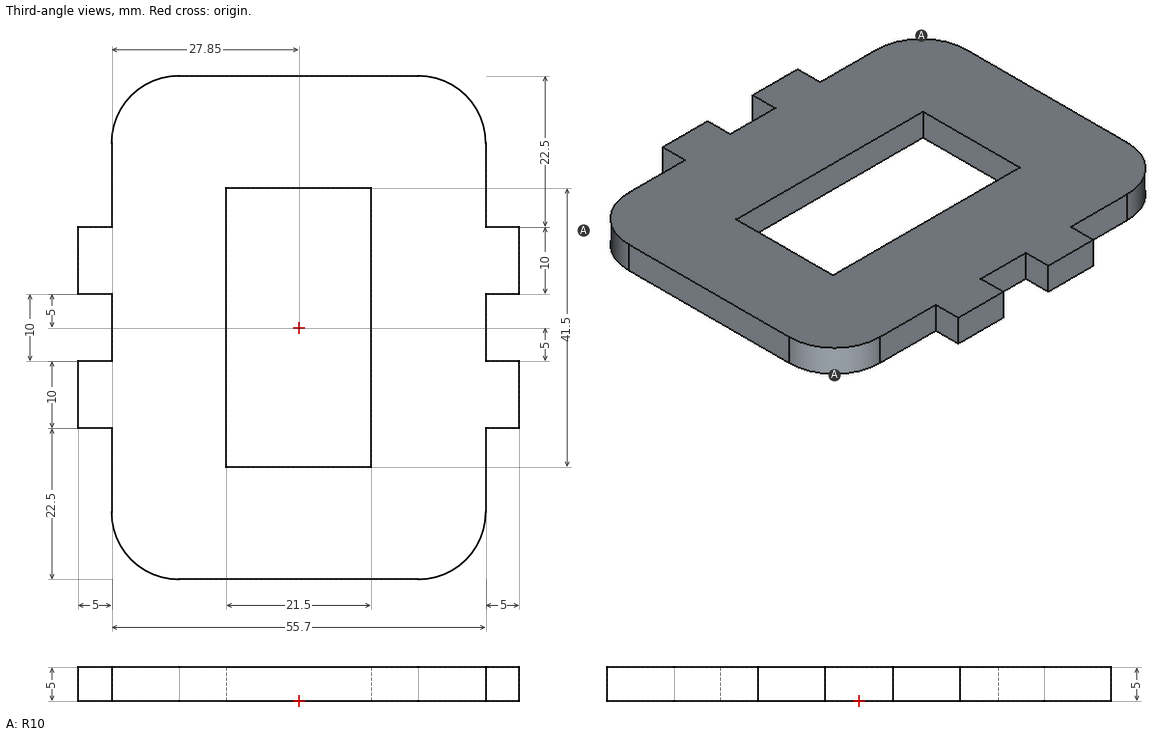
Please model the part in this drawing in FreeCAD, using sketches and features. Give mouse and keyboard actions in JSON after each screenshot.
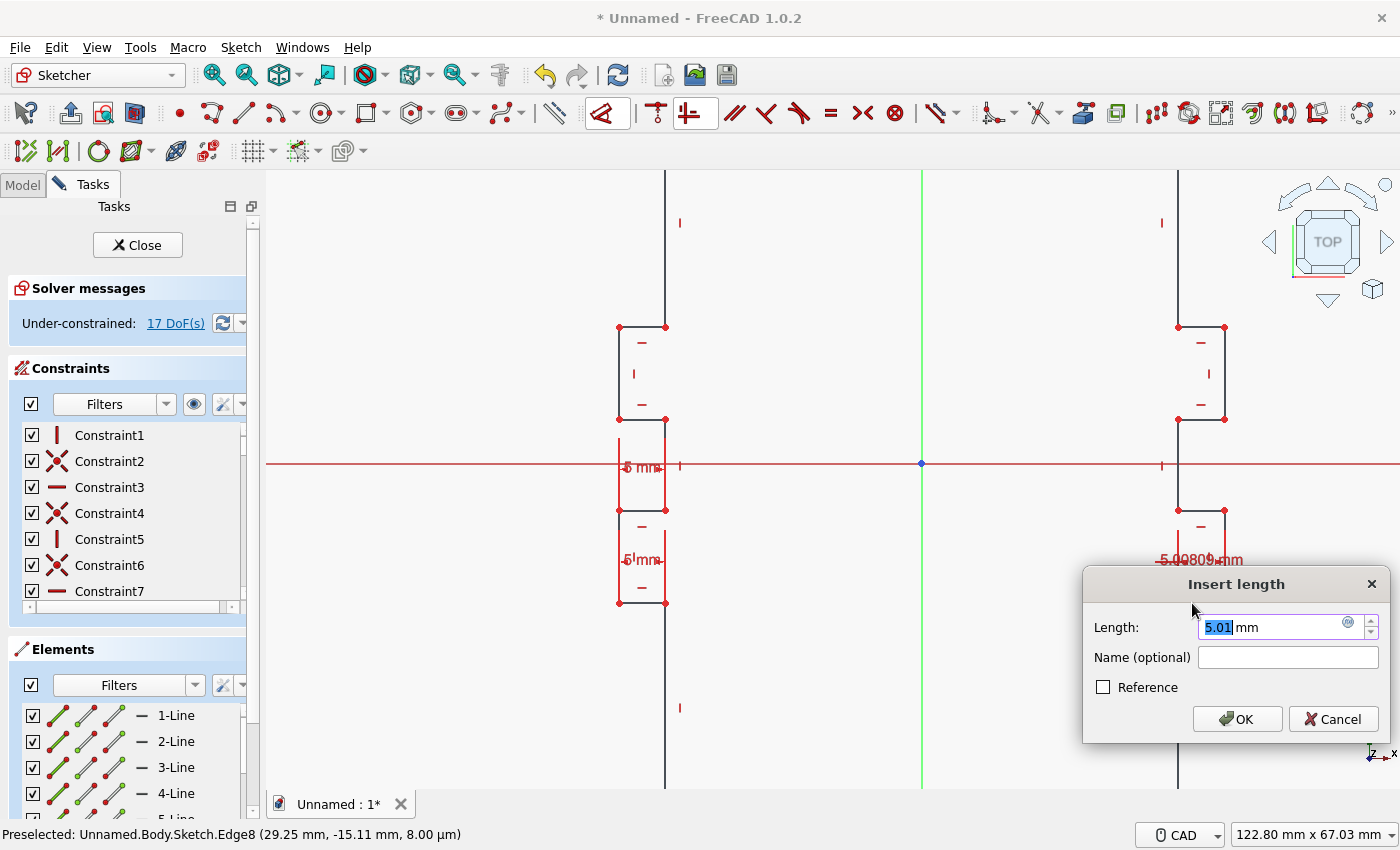
{"action": "type", "text": "5"}
{"action": "key", "text": "Return"}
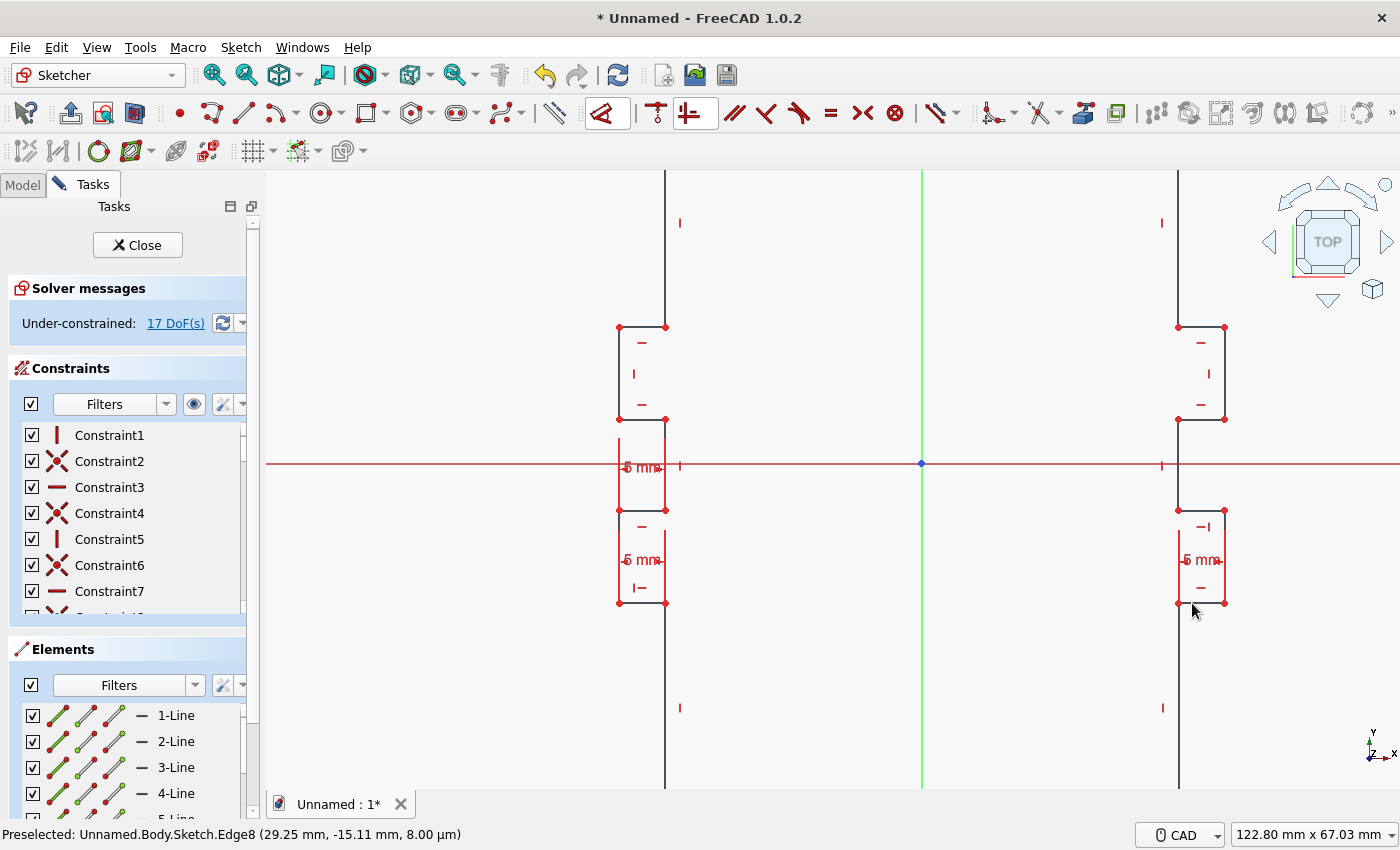
{"action": "left_click", "coordinate": [1211, 511]}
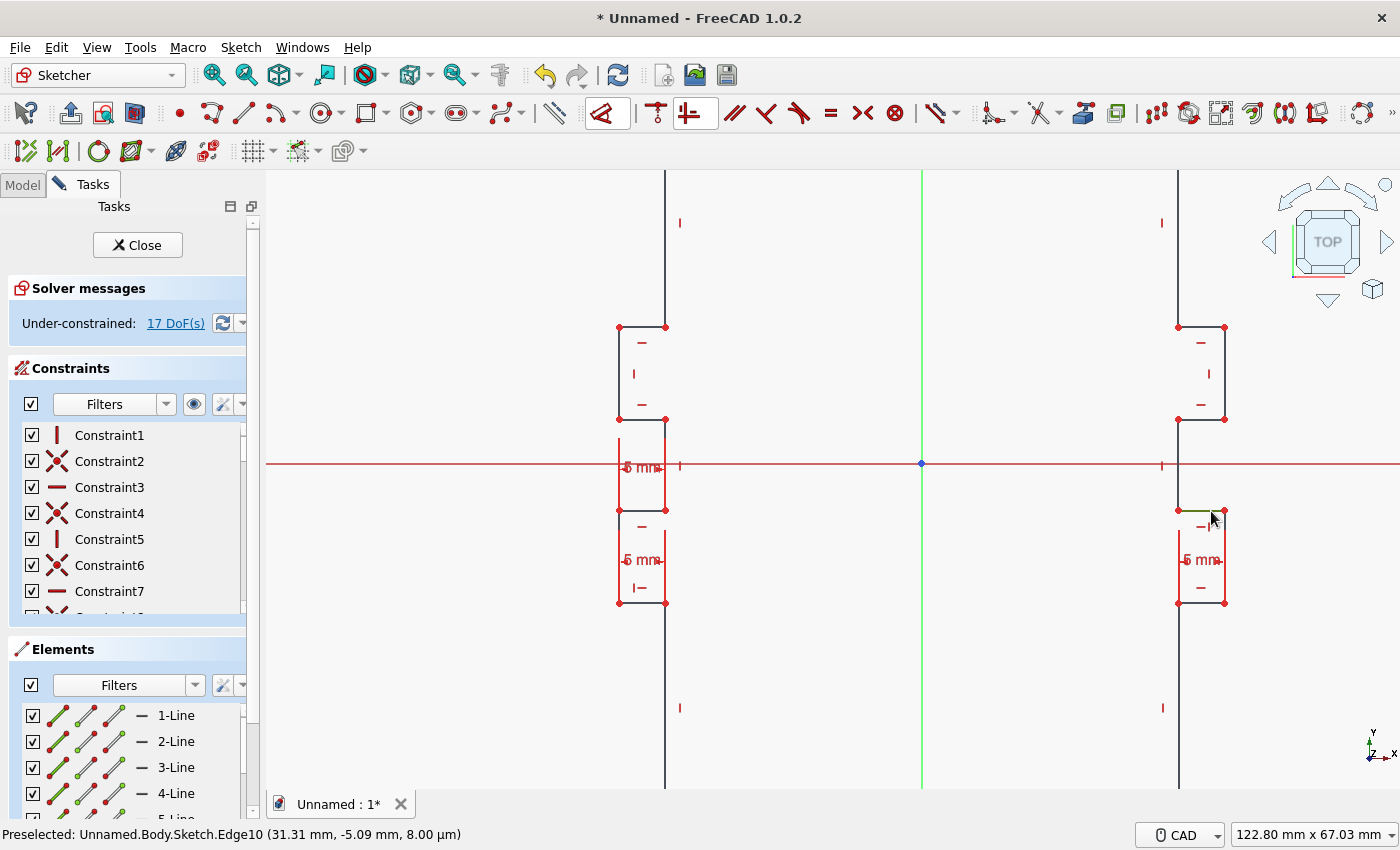
{"action": "left_click", "coordinate": [624, 114]}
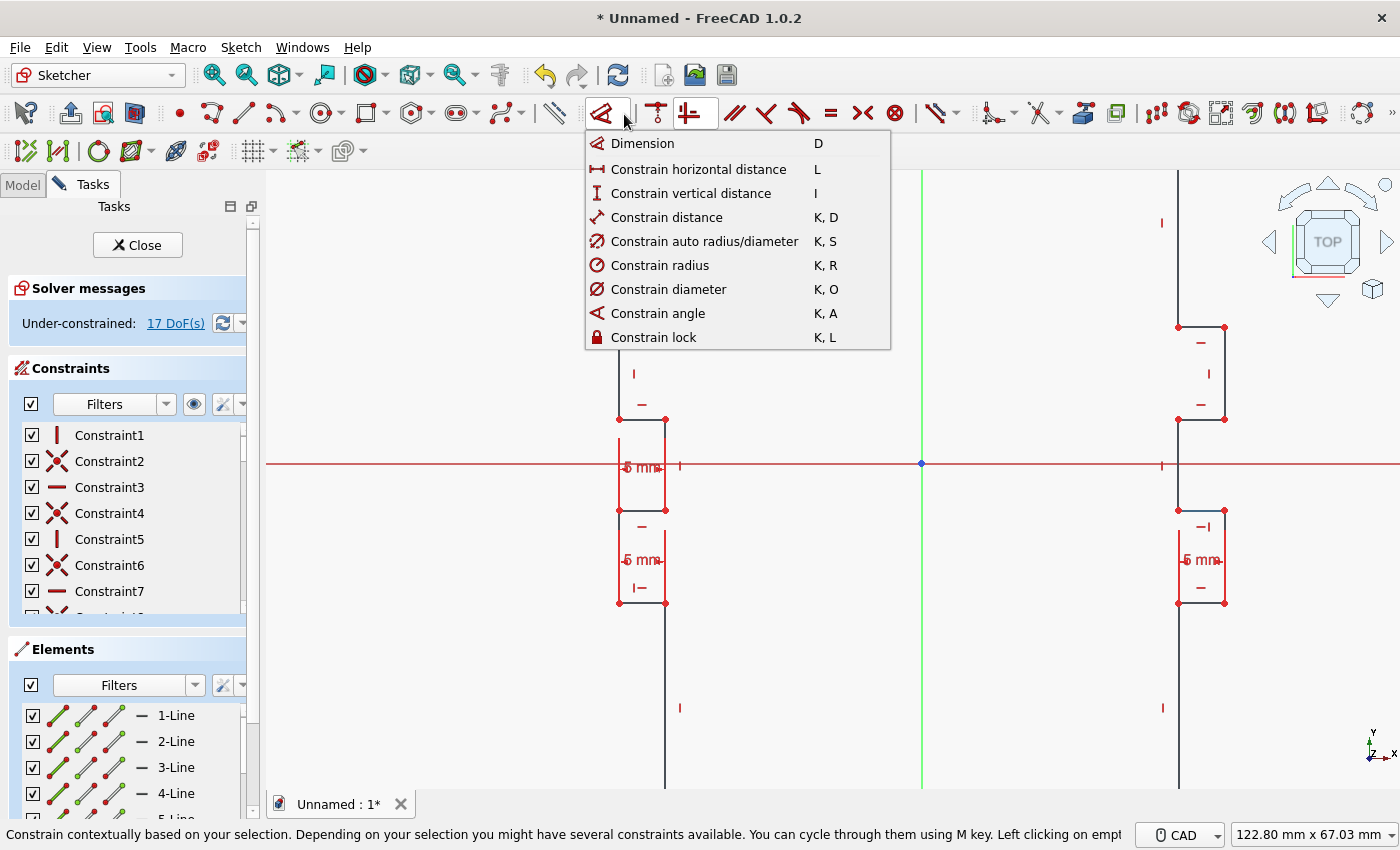
{"action": "left_click", "coordinate": [738, 169]}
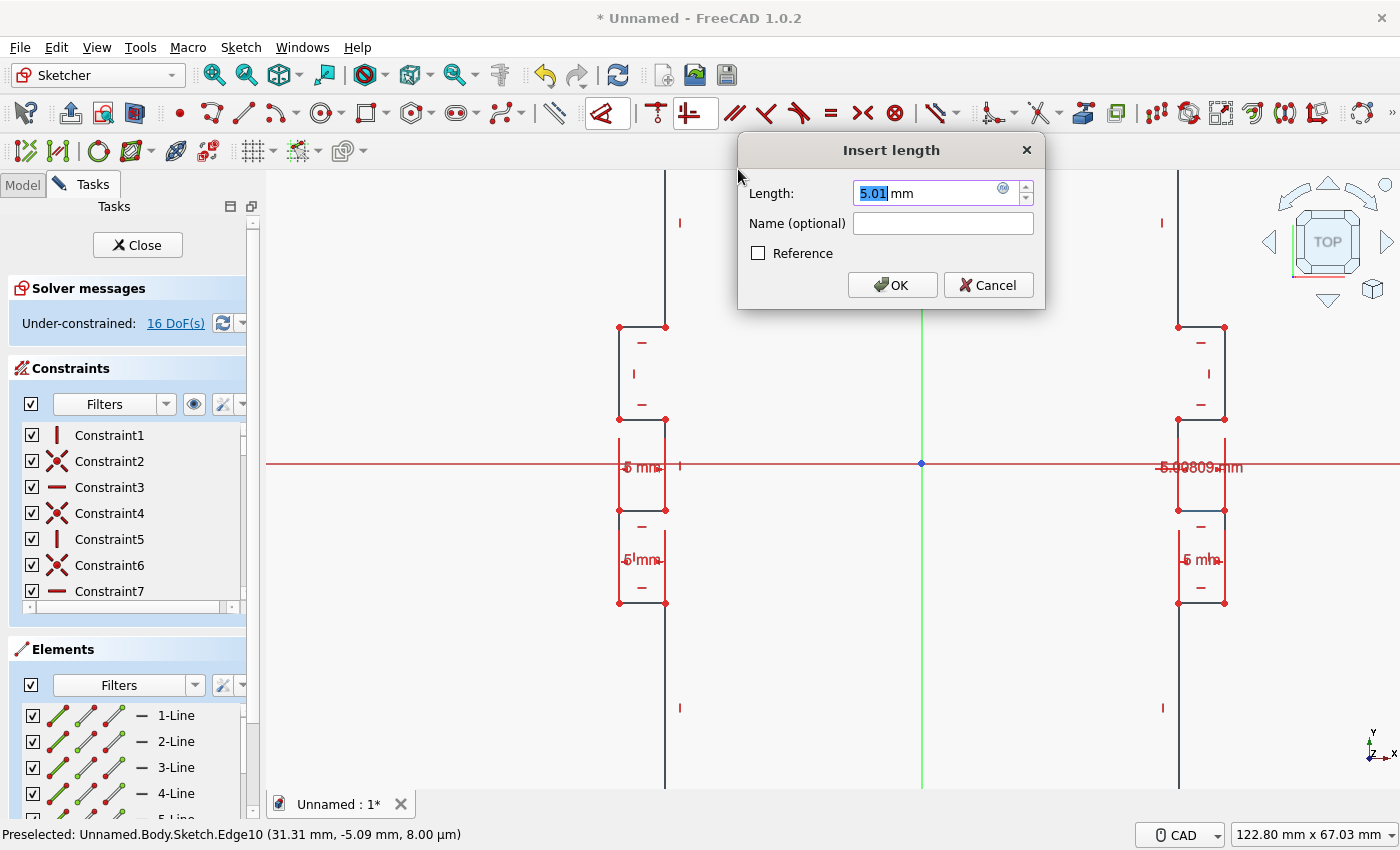
{"action": "type", "text": "5"}
{"action": "key", "text": "Return"}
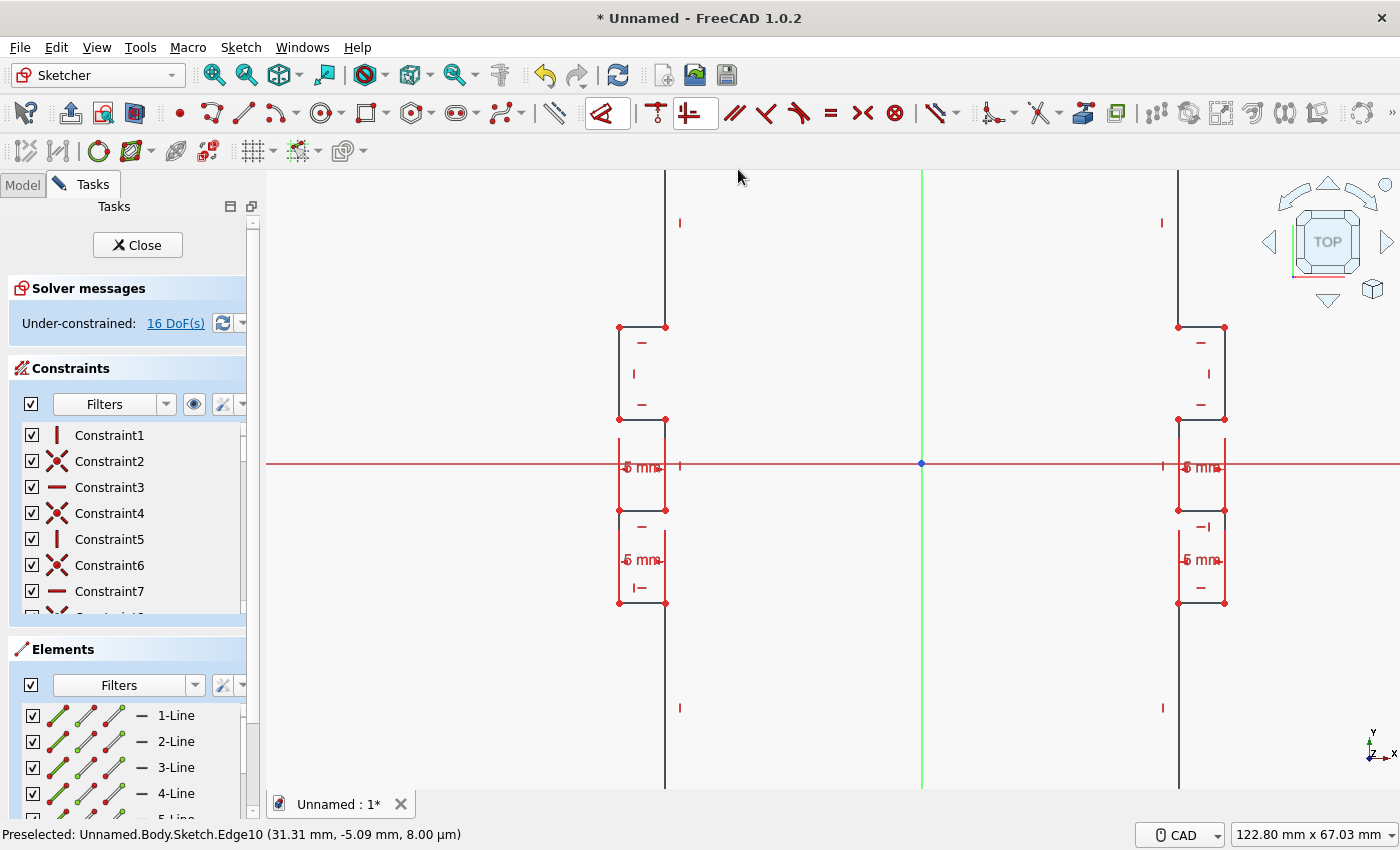
{"action": "left_click", "coordinate": [1192, 420]}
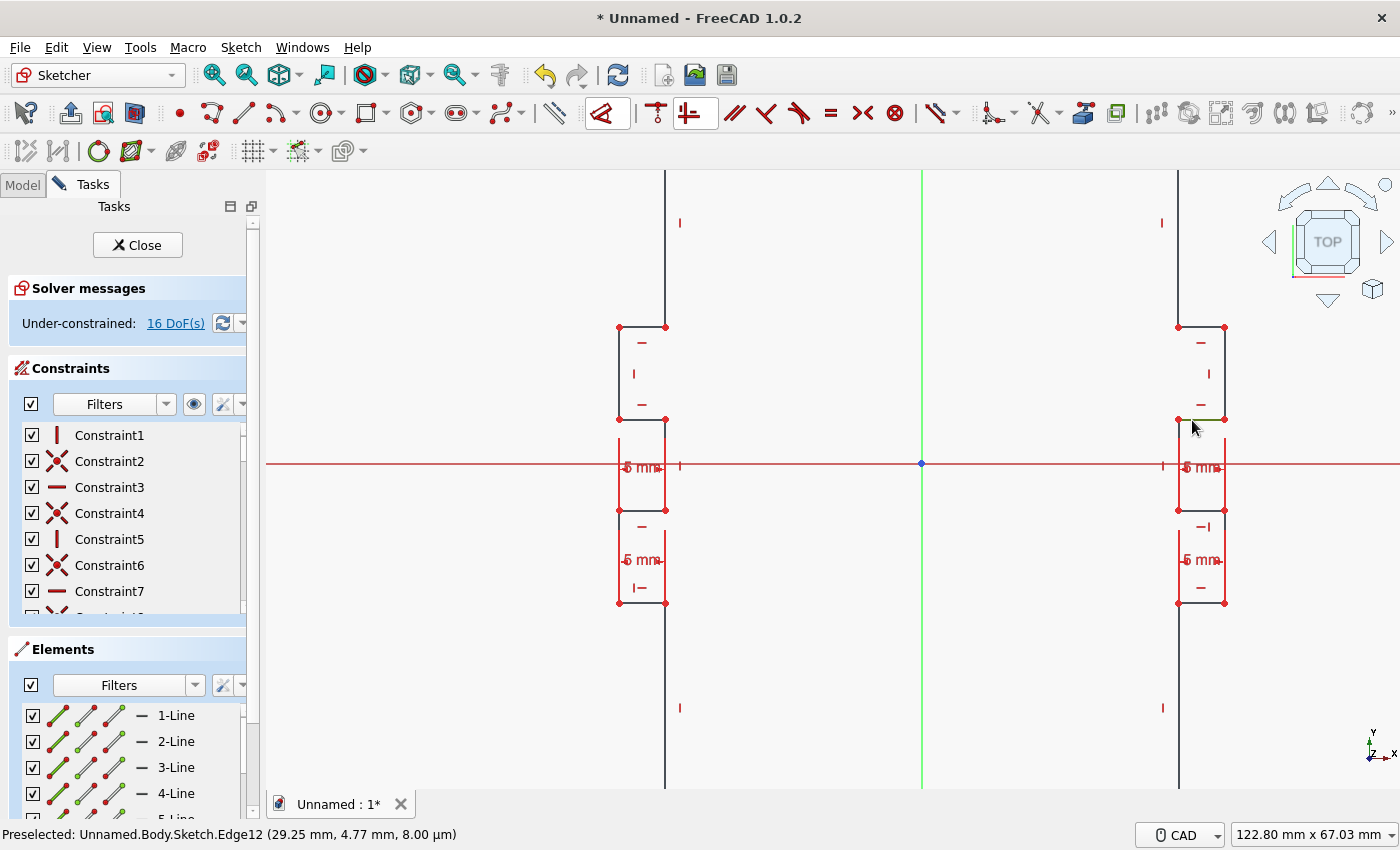
{"action": "left_click", "coordinate": [624, 114]}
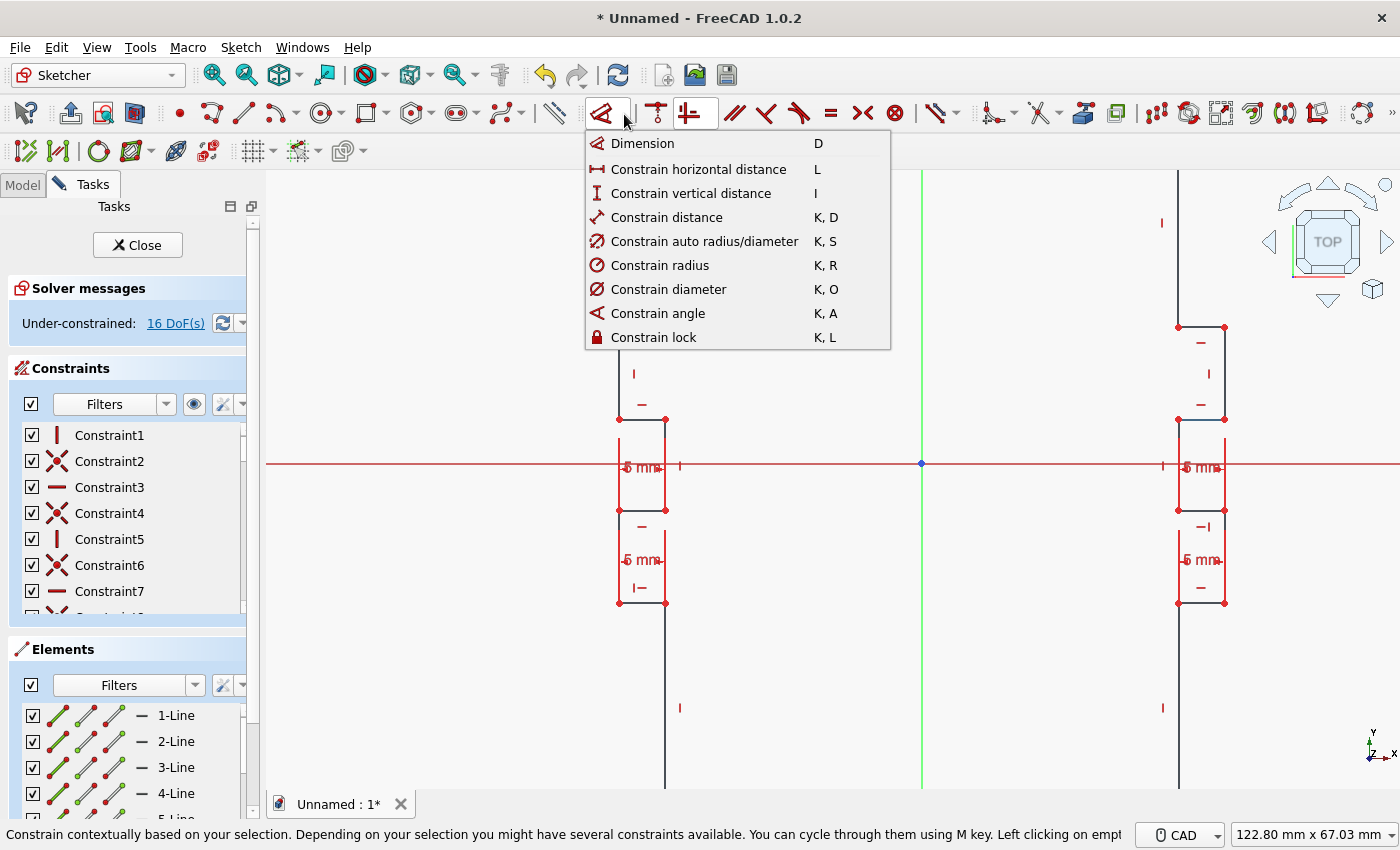
{"action": "left_click", "coordinate": [738, 169]}